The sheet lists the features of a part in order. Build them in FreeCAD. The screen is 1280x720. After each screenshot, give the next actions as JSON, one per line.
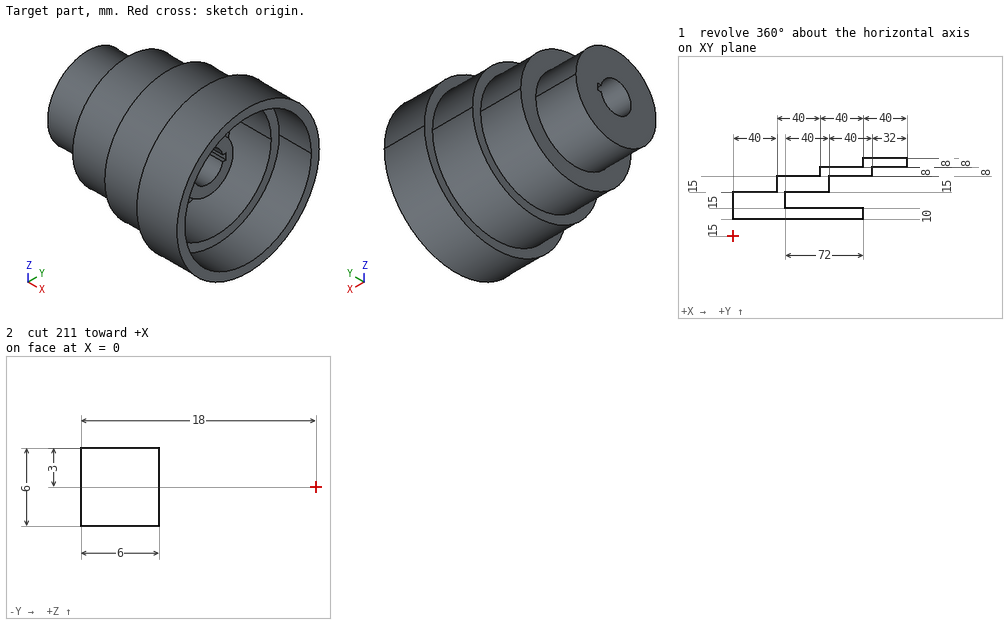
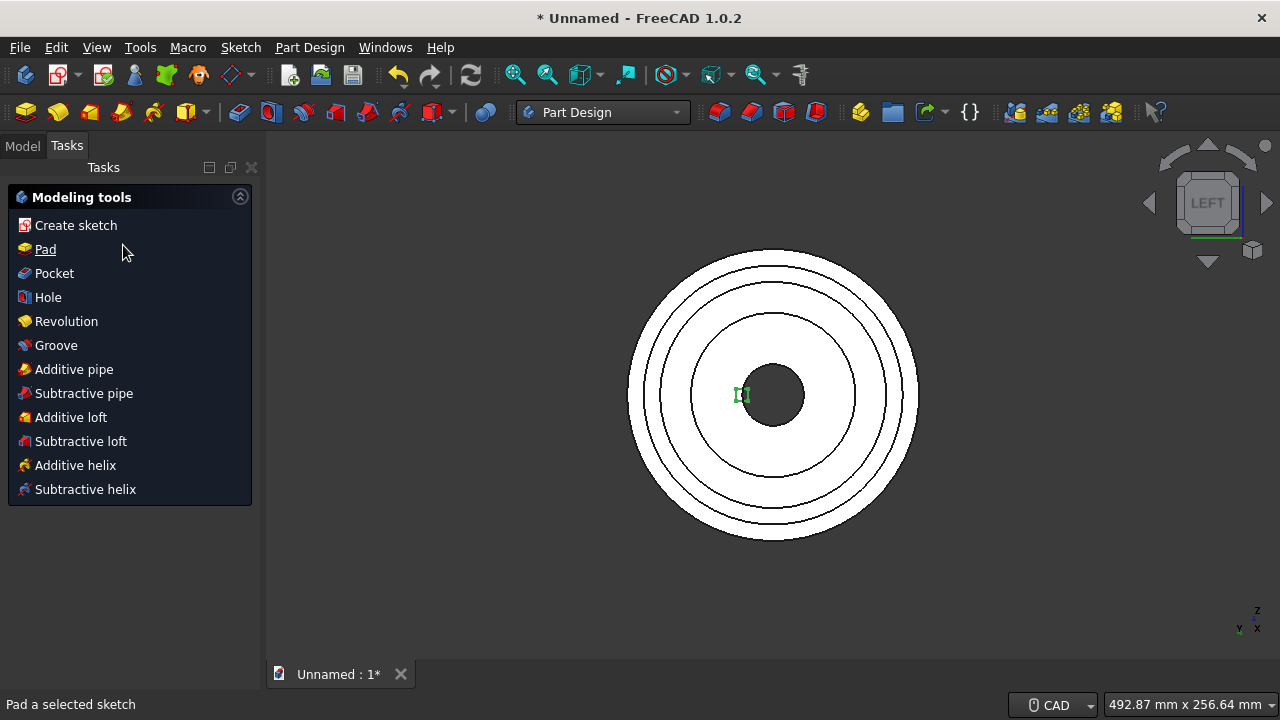
{"action": "left_click", "coordinate": [240, 112]}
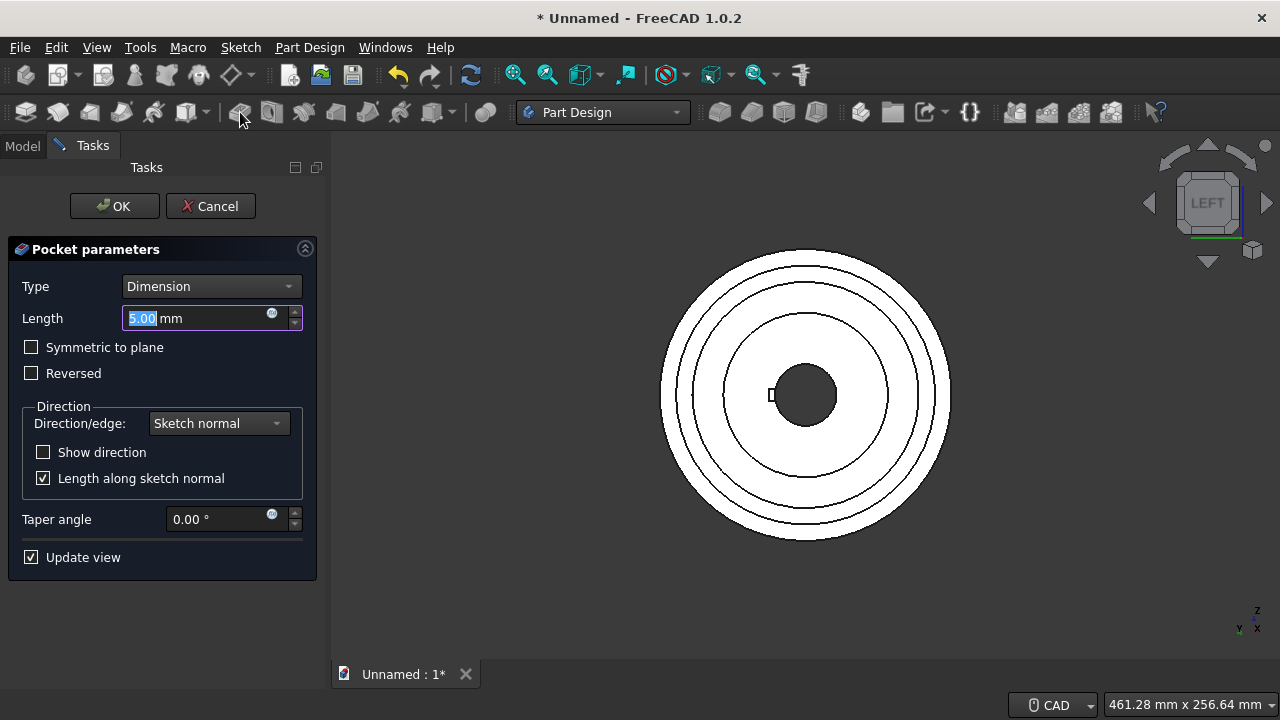
{"action": "type", "text": "211"}
{"action": "key", "text": "Tab"}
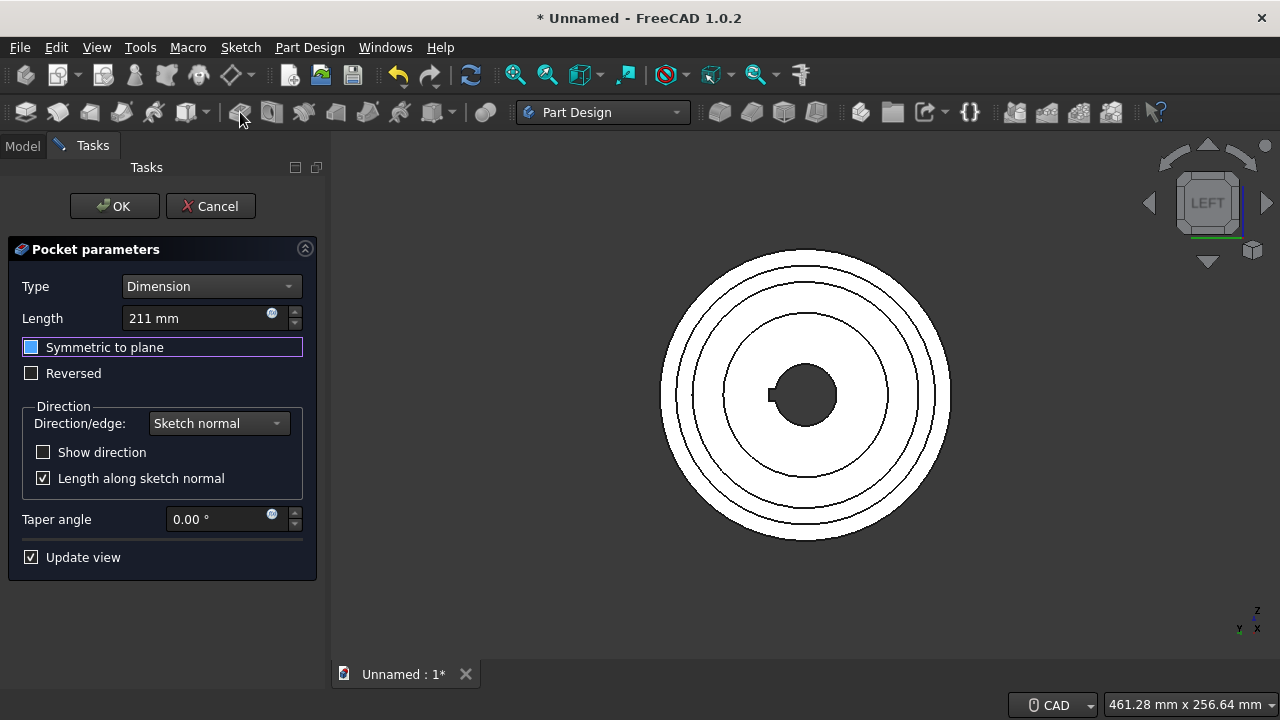
{"action": "left_click", "coordinate": [115, 206]}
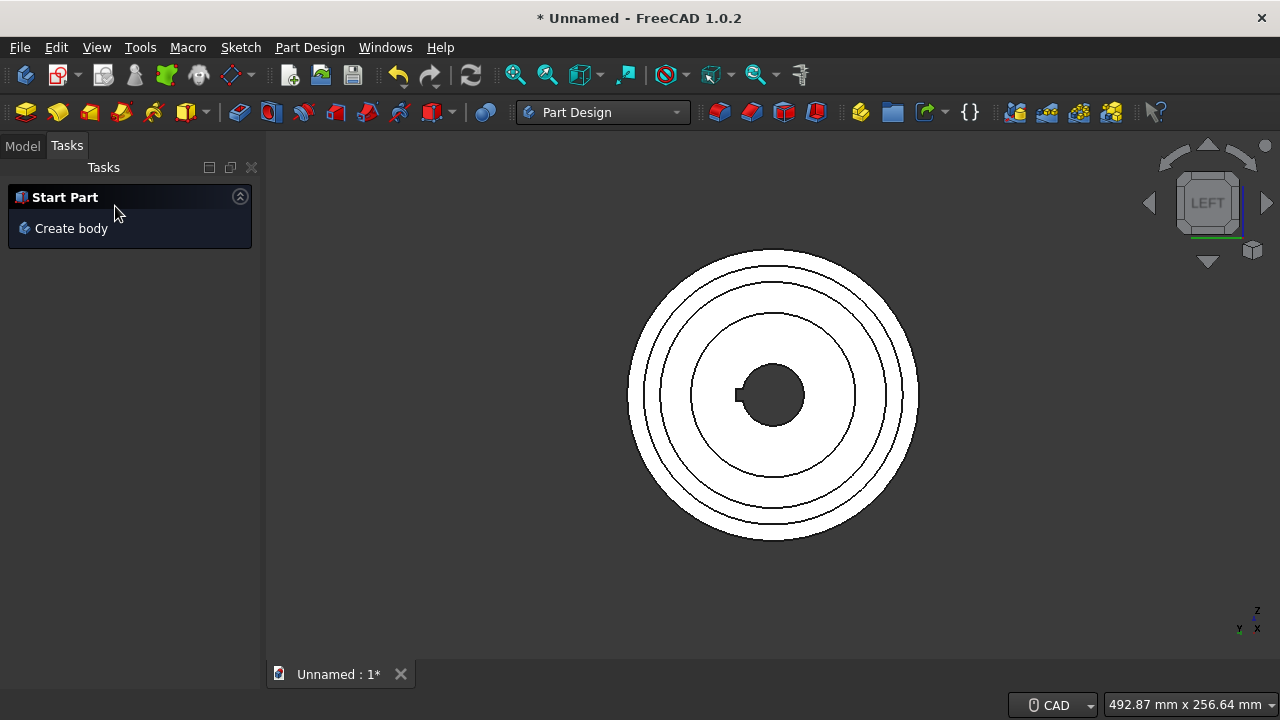
{"action": "key", "text": "0"}